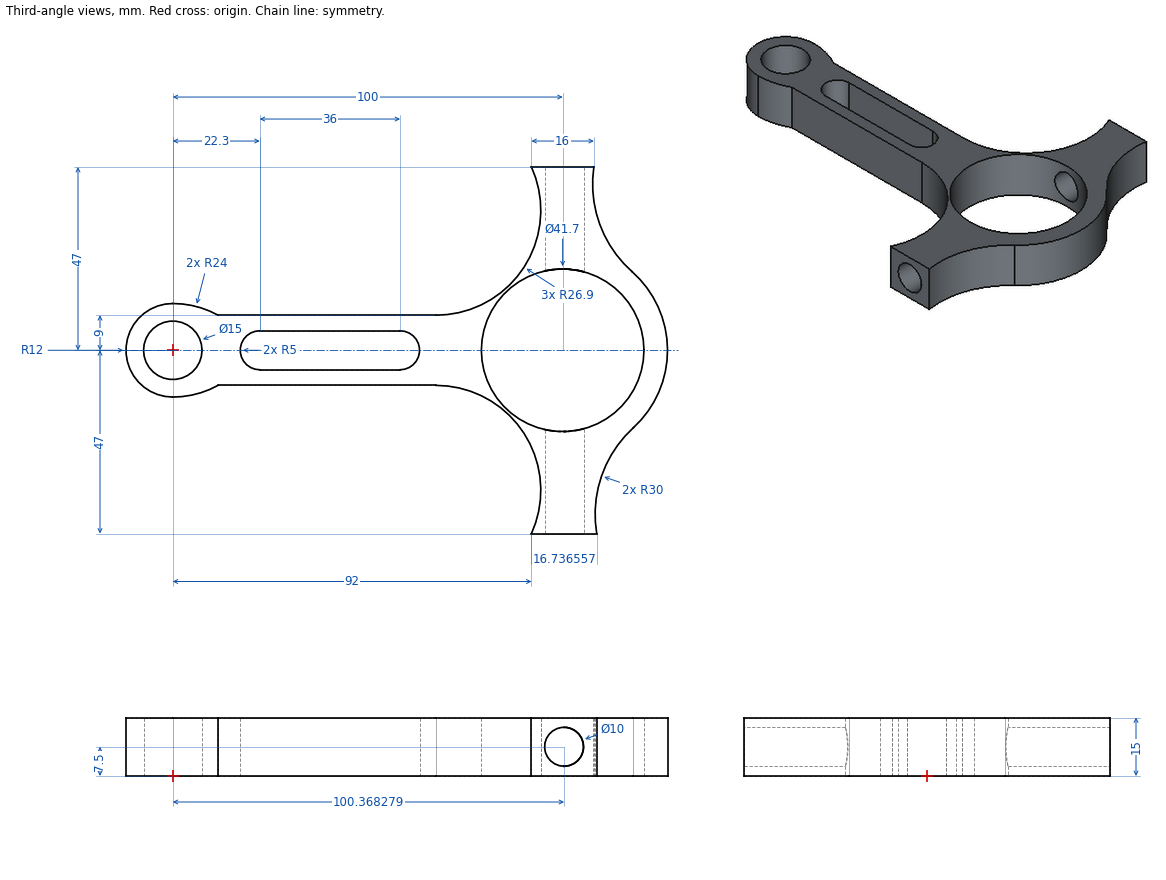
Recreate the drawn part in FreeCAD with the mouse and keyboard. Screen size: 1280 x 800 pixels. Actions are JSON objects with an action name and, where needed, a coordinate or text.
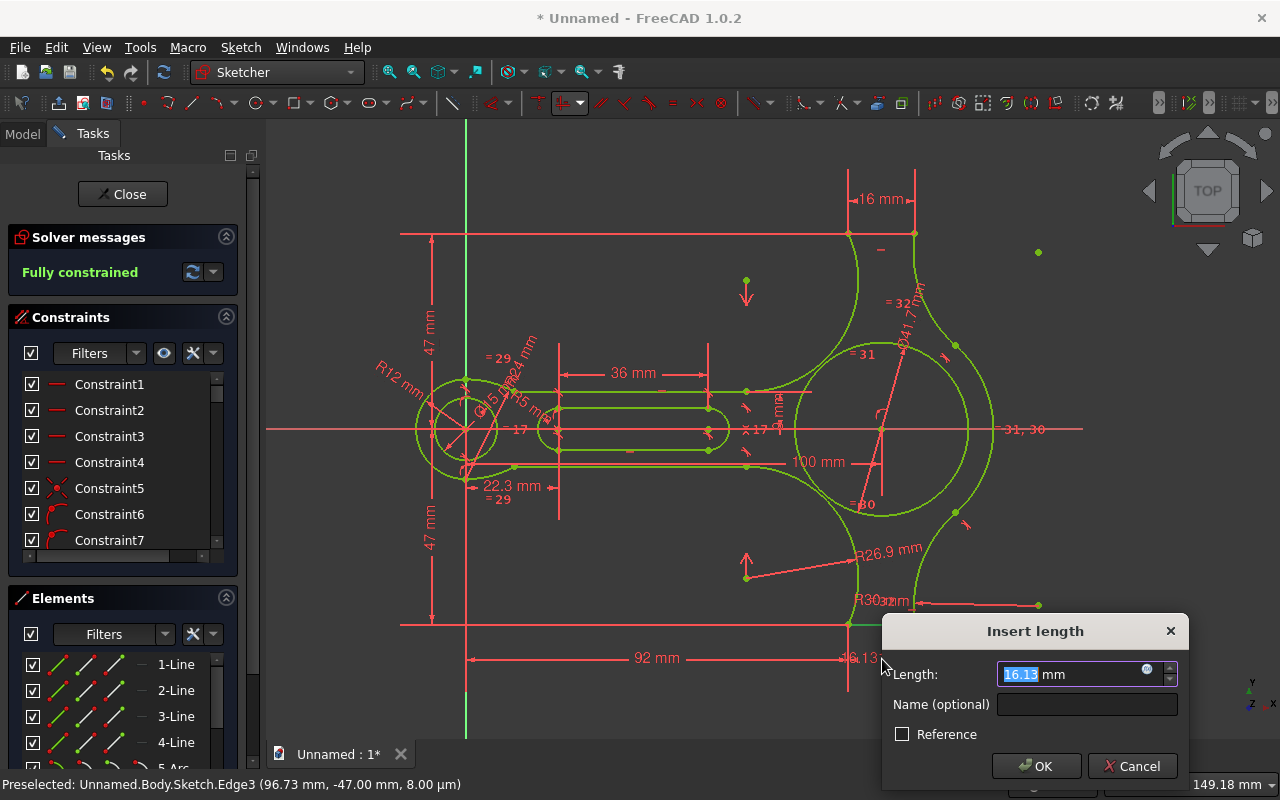
{"action": "type", "text": "16.736557"}
{"action": "key", "text": "Return"}
{"action": "key", "text": "Escape"}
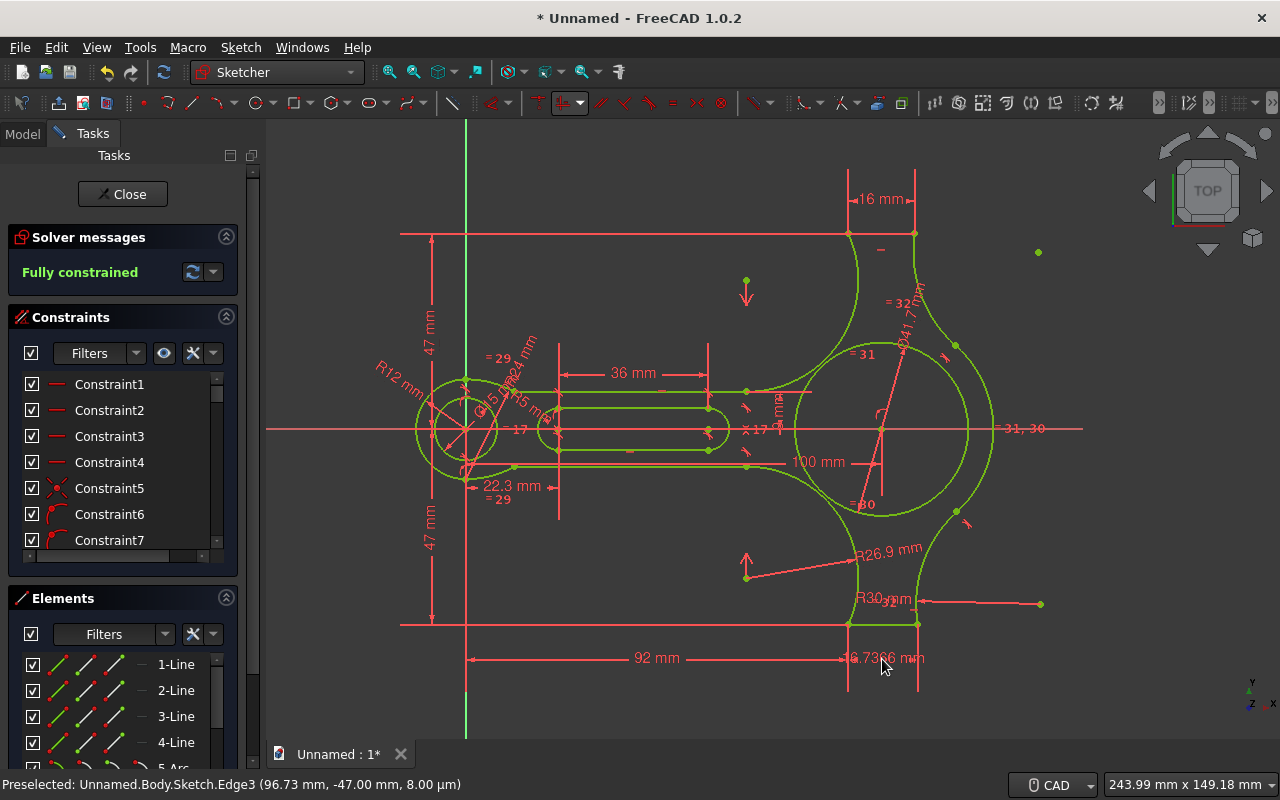
{"action": "left_click", "coordinate": [123, 194]}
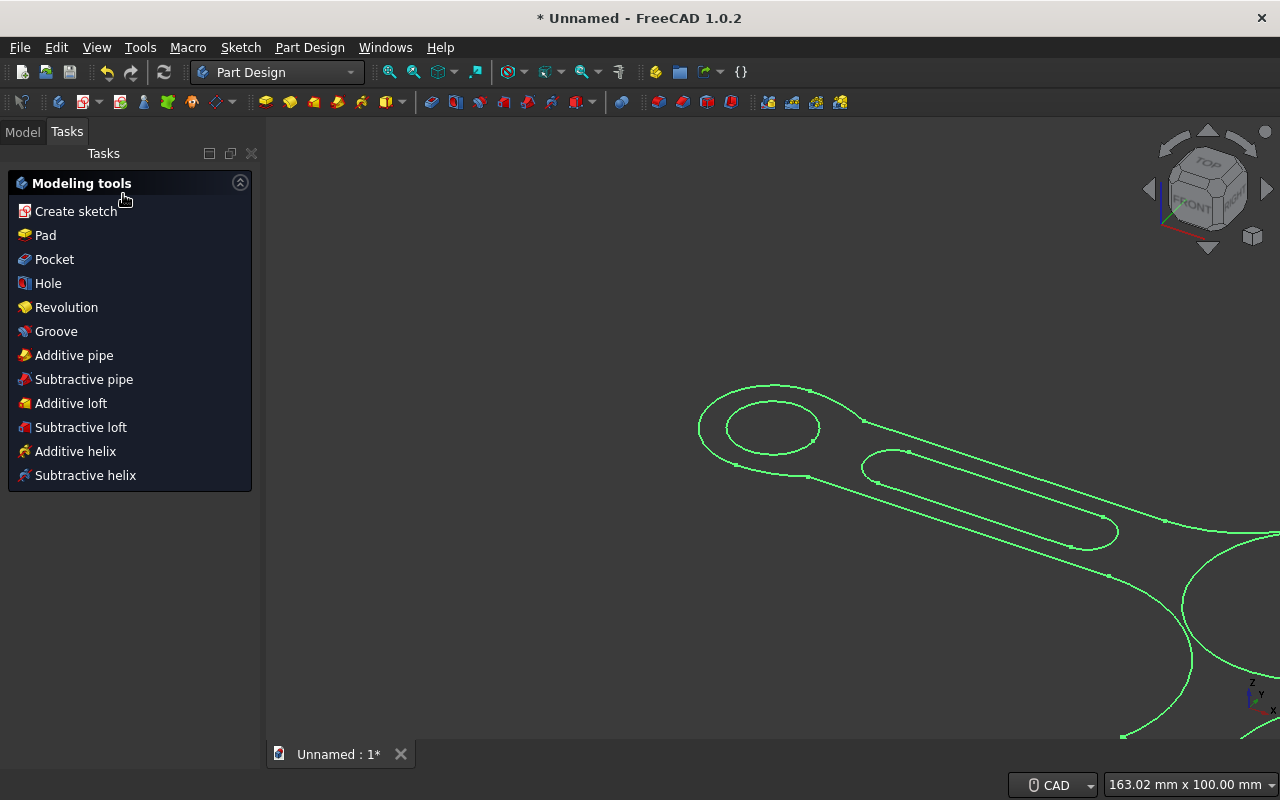
{"action": "left_click", "coordinate": [266, 102]}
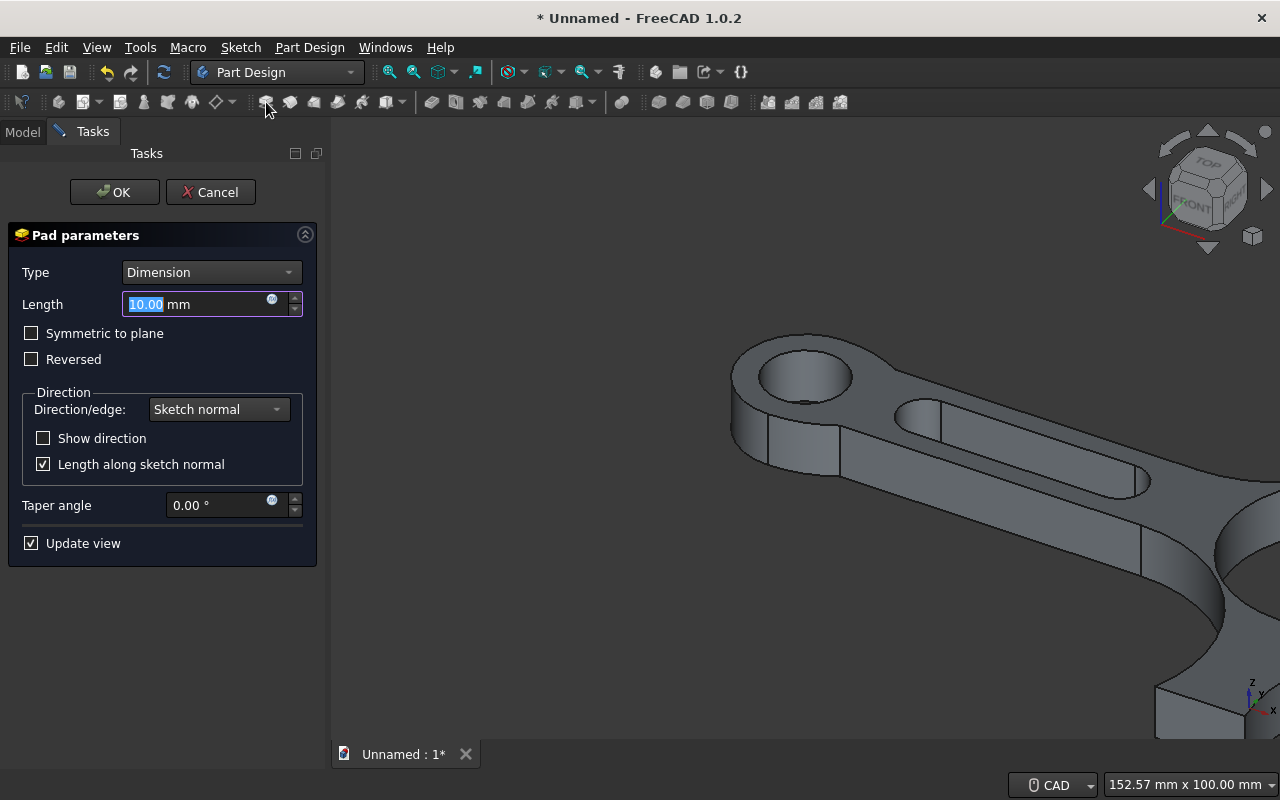
{"action": "type", "text": "15"}
{"action": "key", "text": "Tab"}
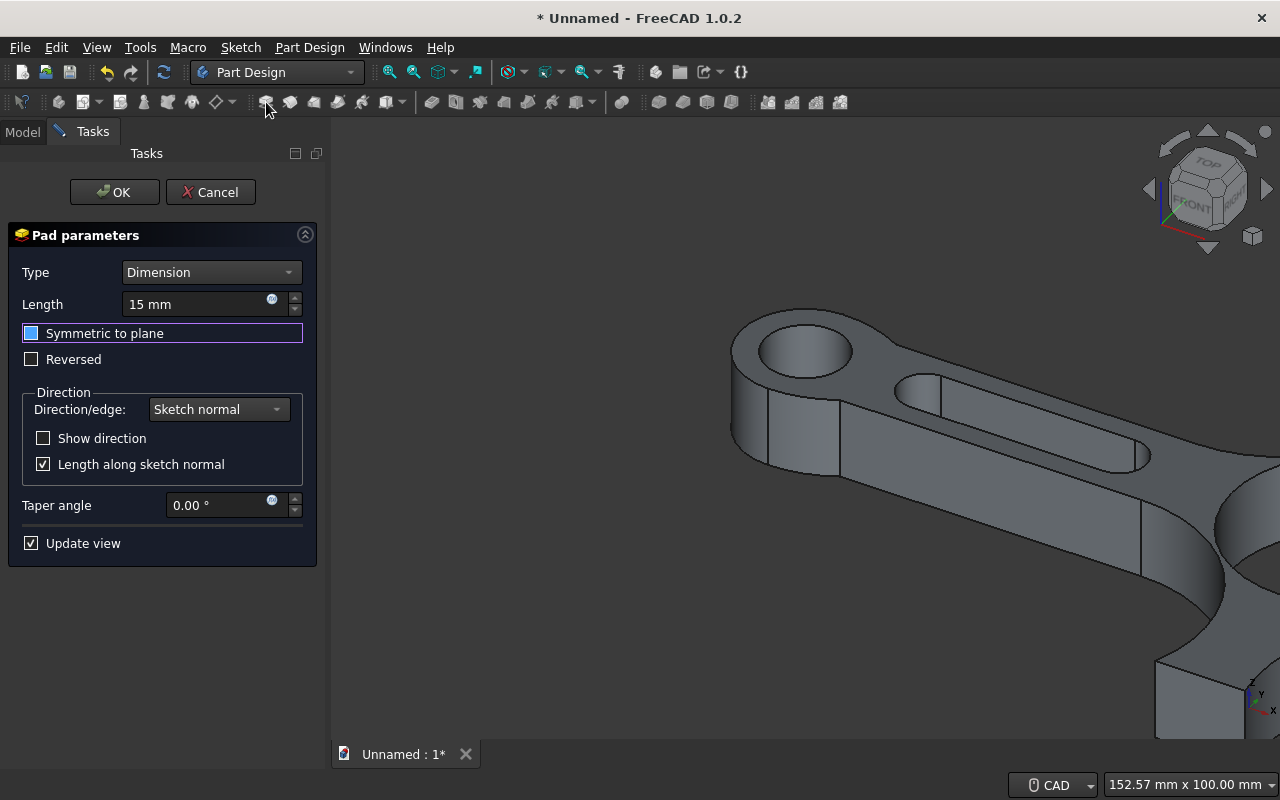
{"action": "left_click", "coordinate": [115, 192]}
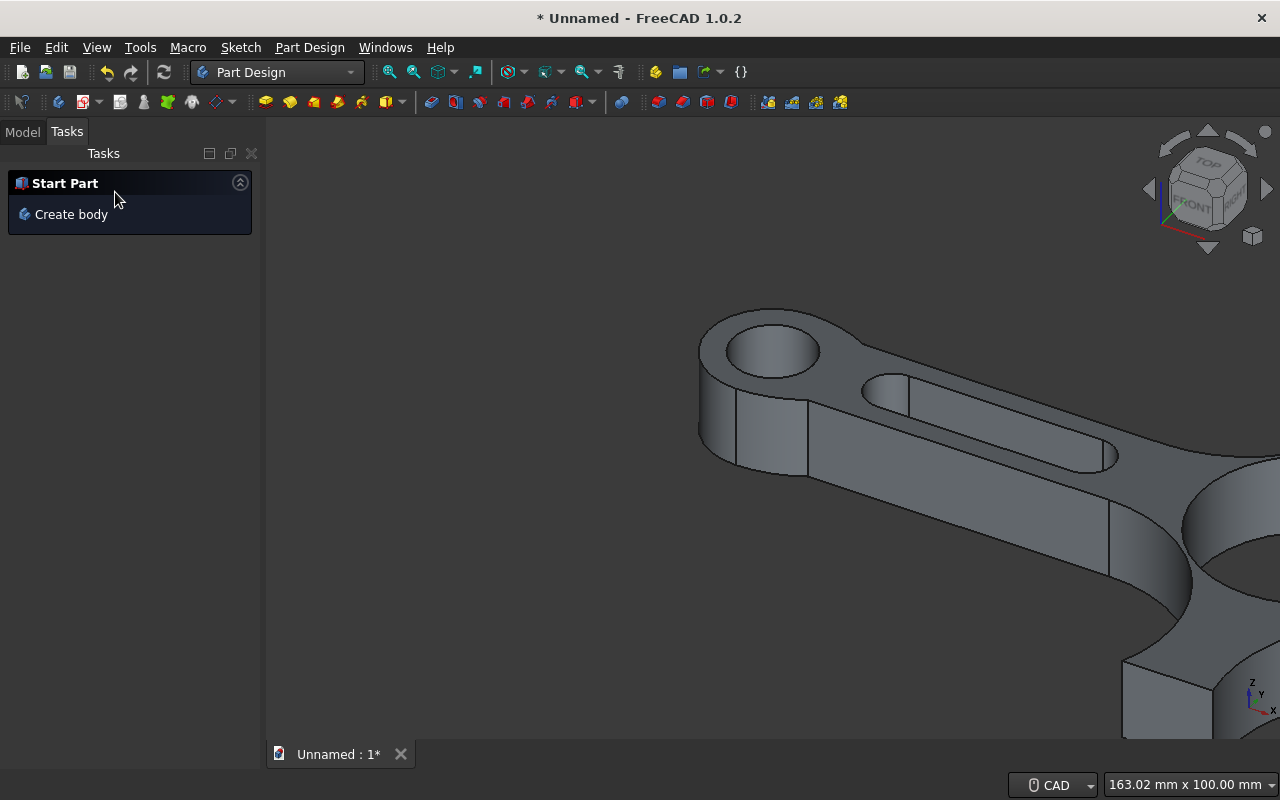
{"action": "left_click", "coordinate": [390, 72]}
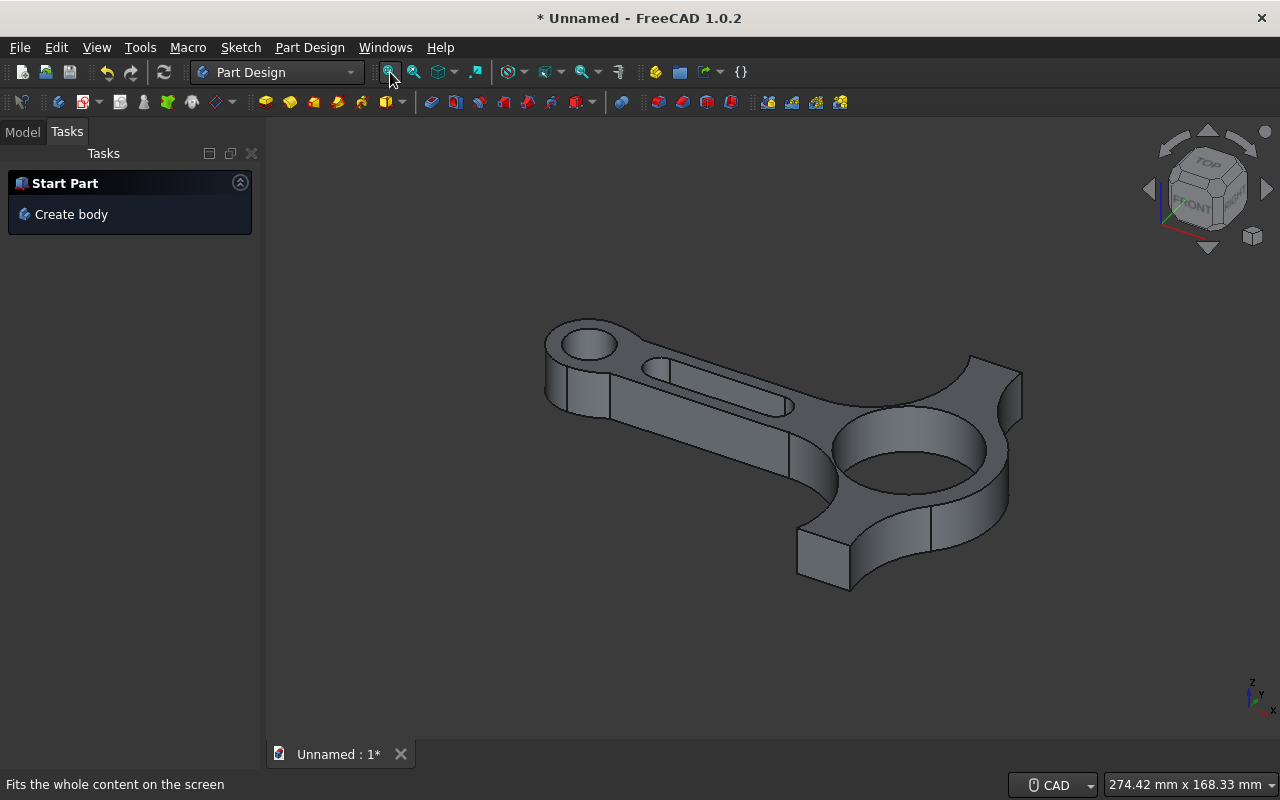
{"action": "left_click", "coordinate": [824, 559]}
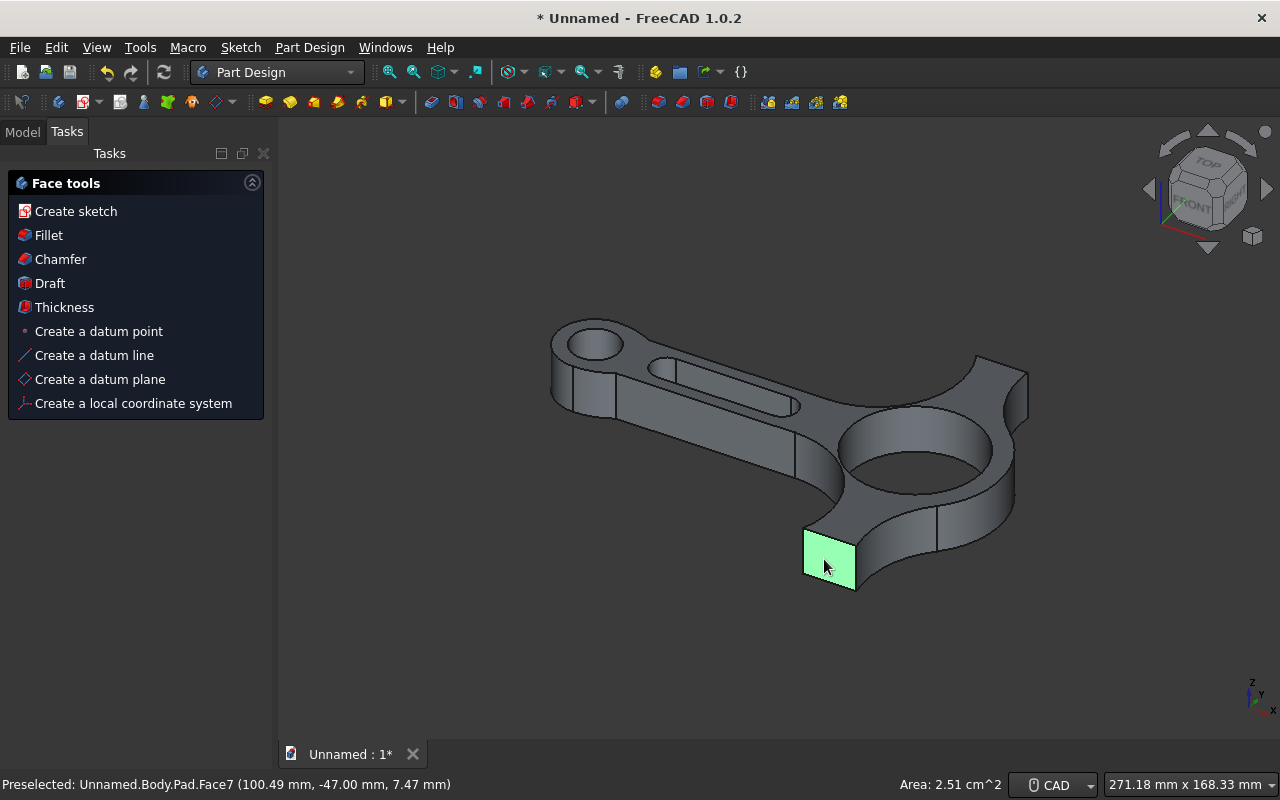
{"action": "left_click", "coordinate": [84, 102]}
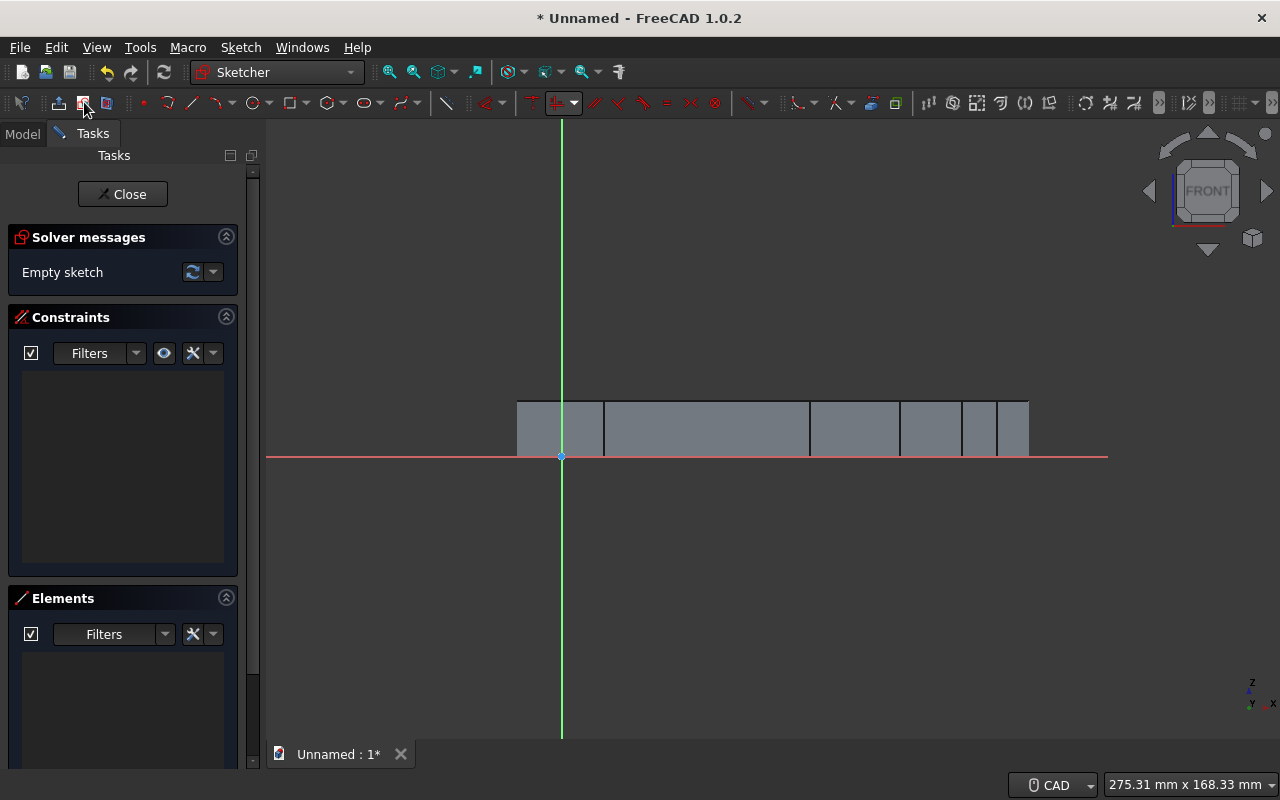
{"action": "scroll", "coordinate": [954, 429], "scroll_direction": "up", "scroll_amount": 12}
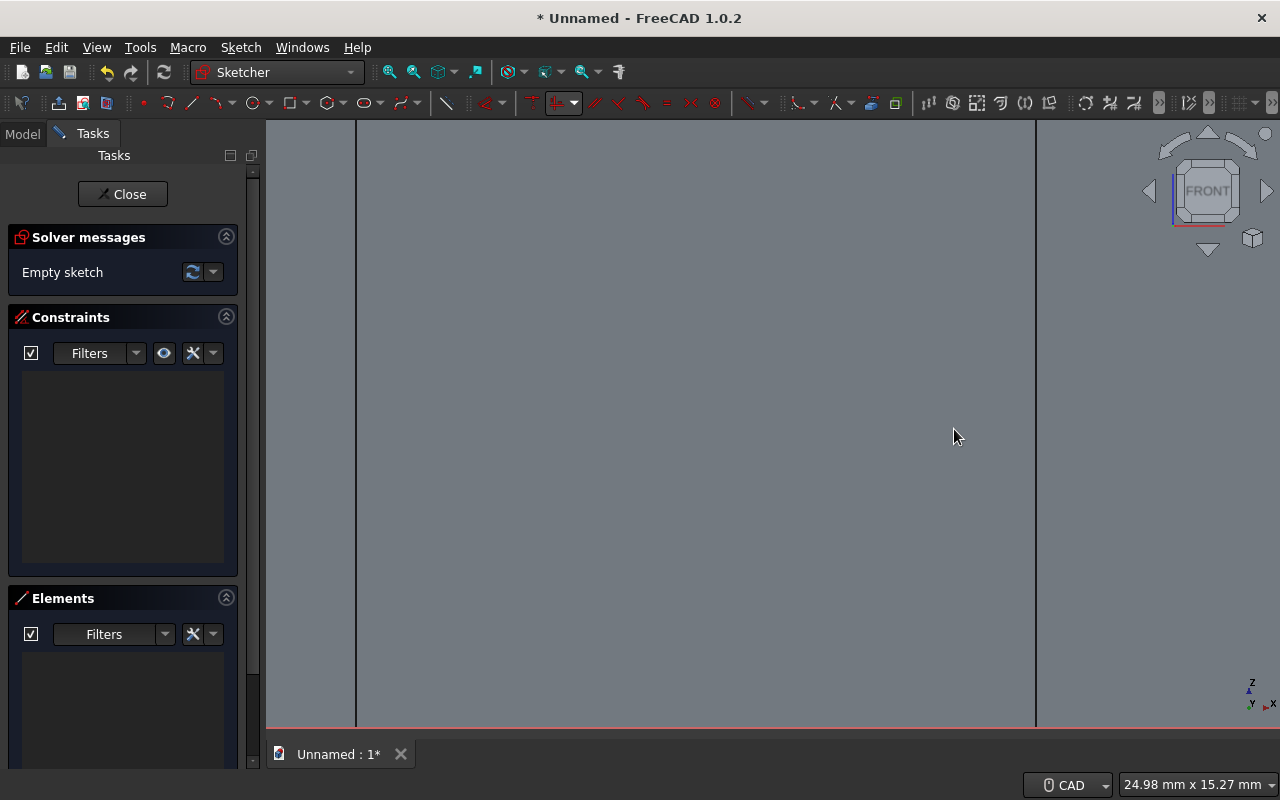
{"action": "left_click", "coordinate": [254, 104]}